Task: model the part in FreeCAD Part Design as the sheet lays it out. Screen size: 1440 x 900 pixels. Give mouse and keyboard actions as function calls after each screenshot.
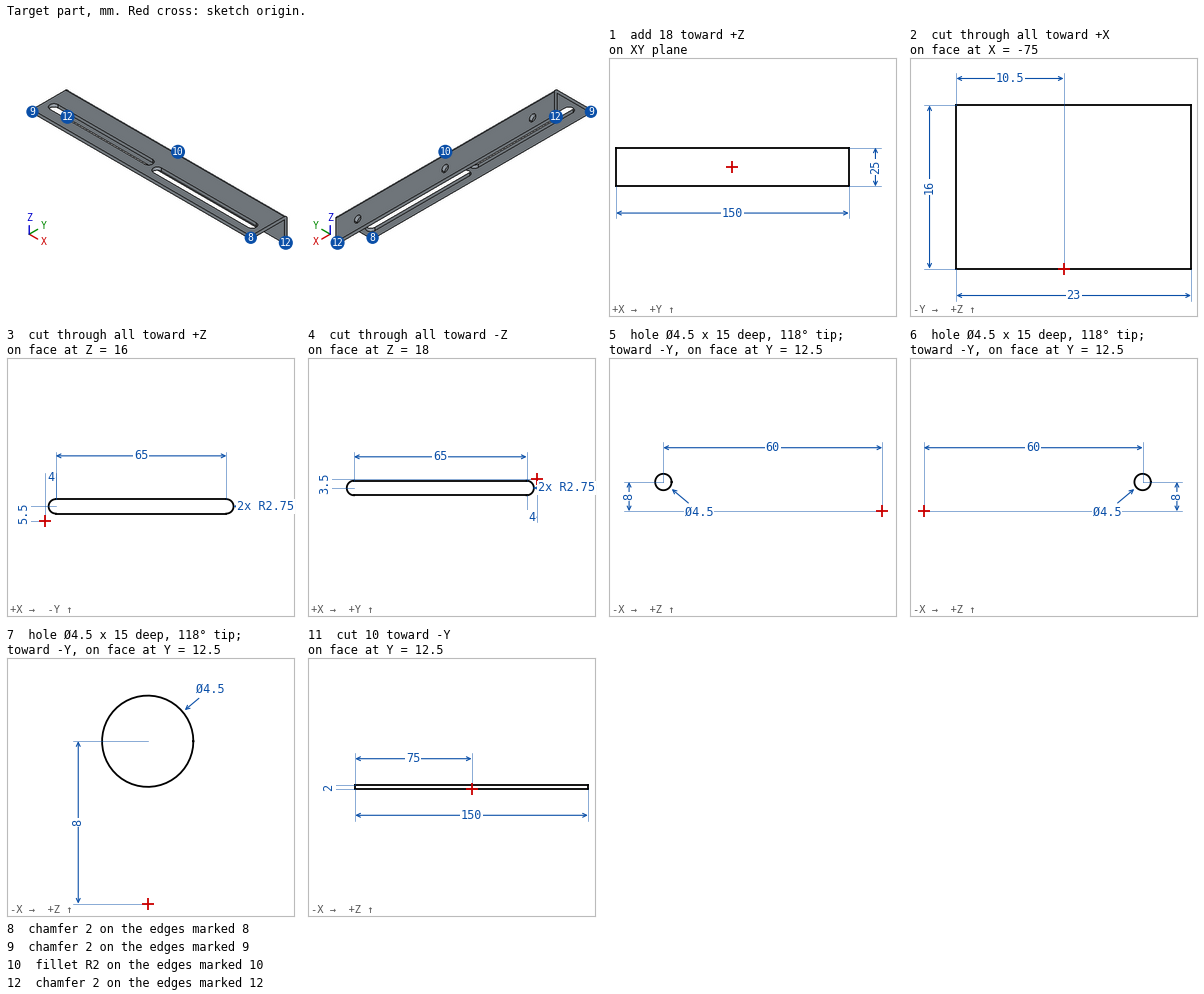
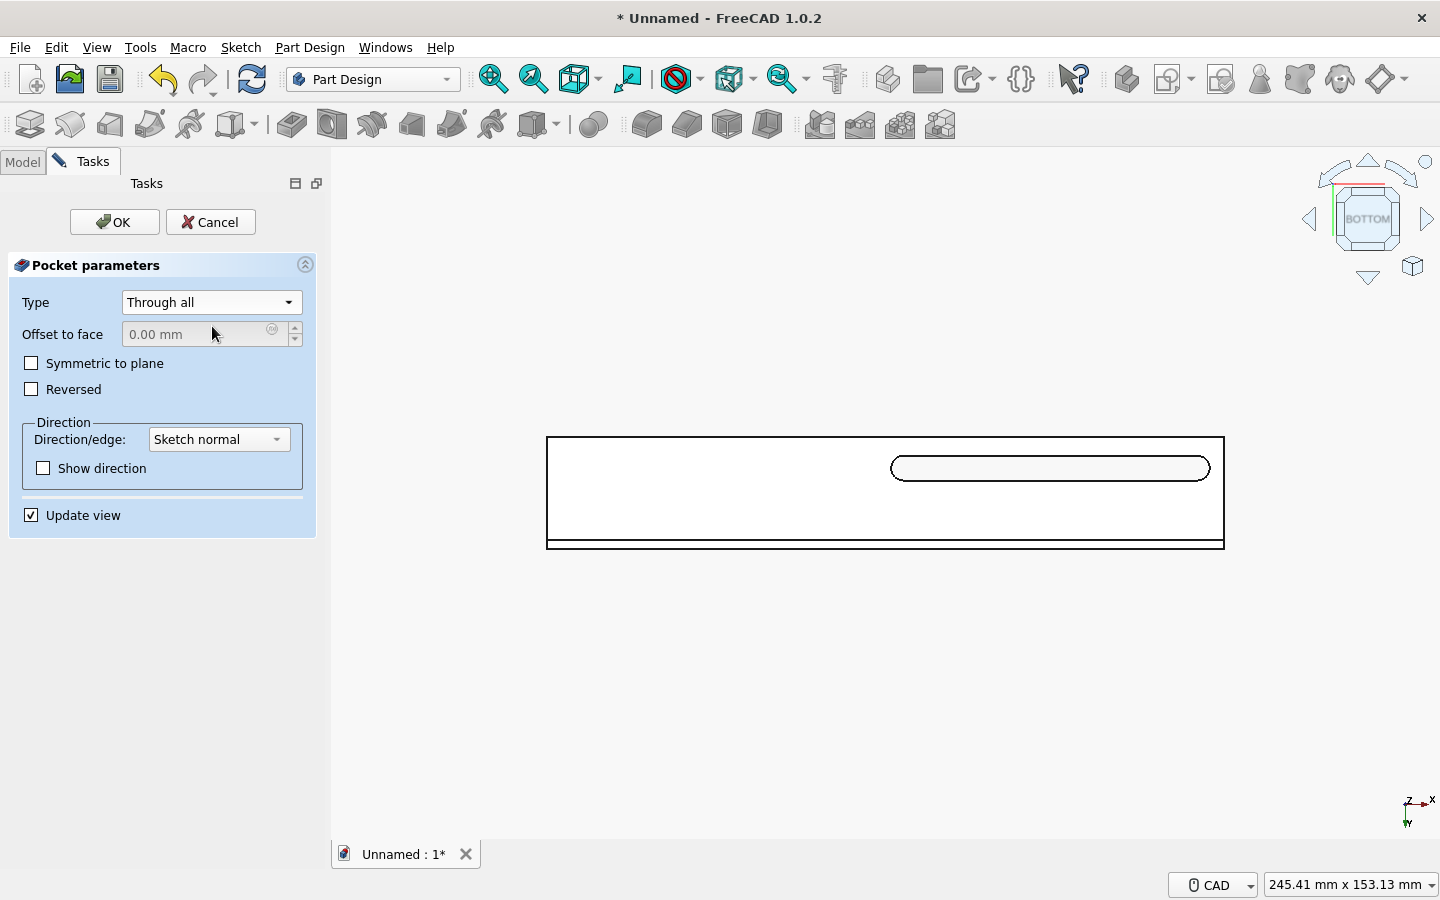
click(115, 222)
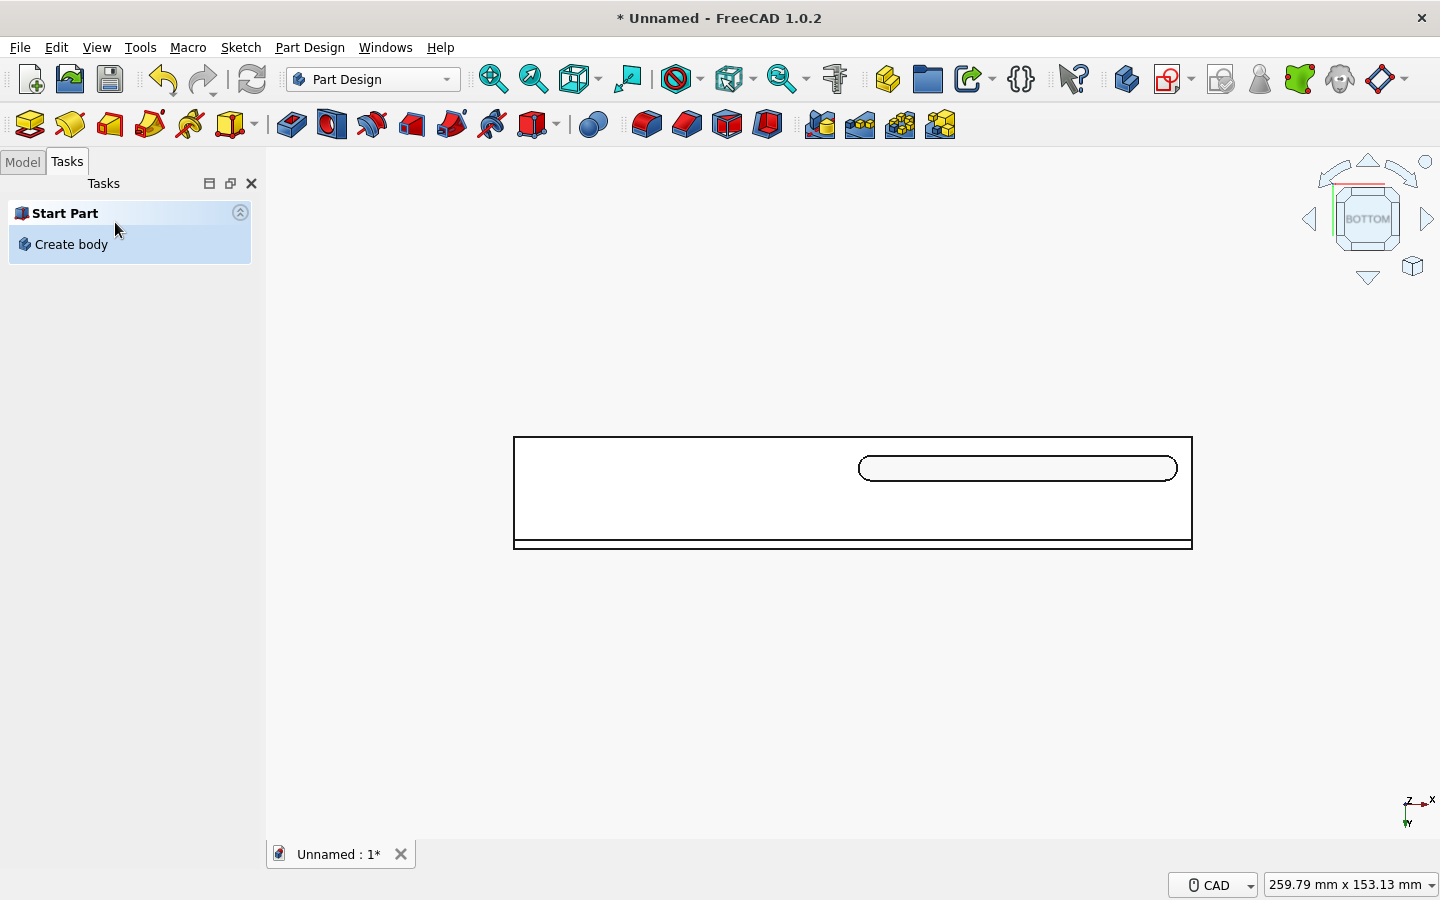
key(0)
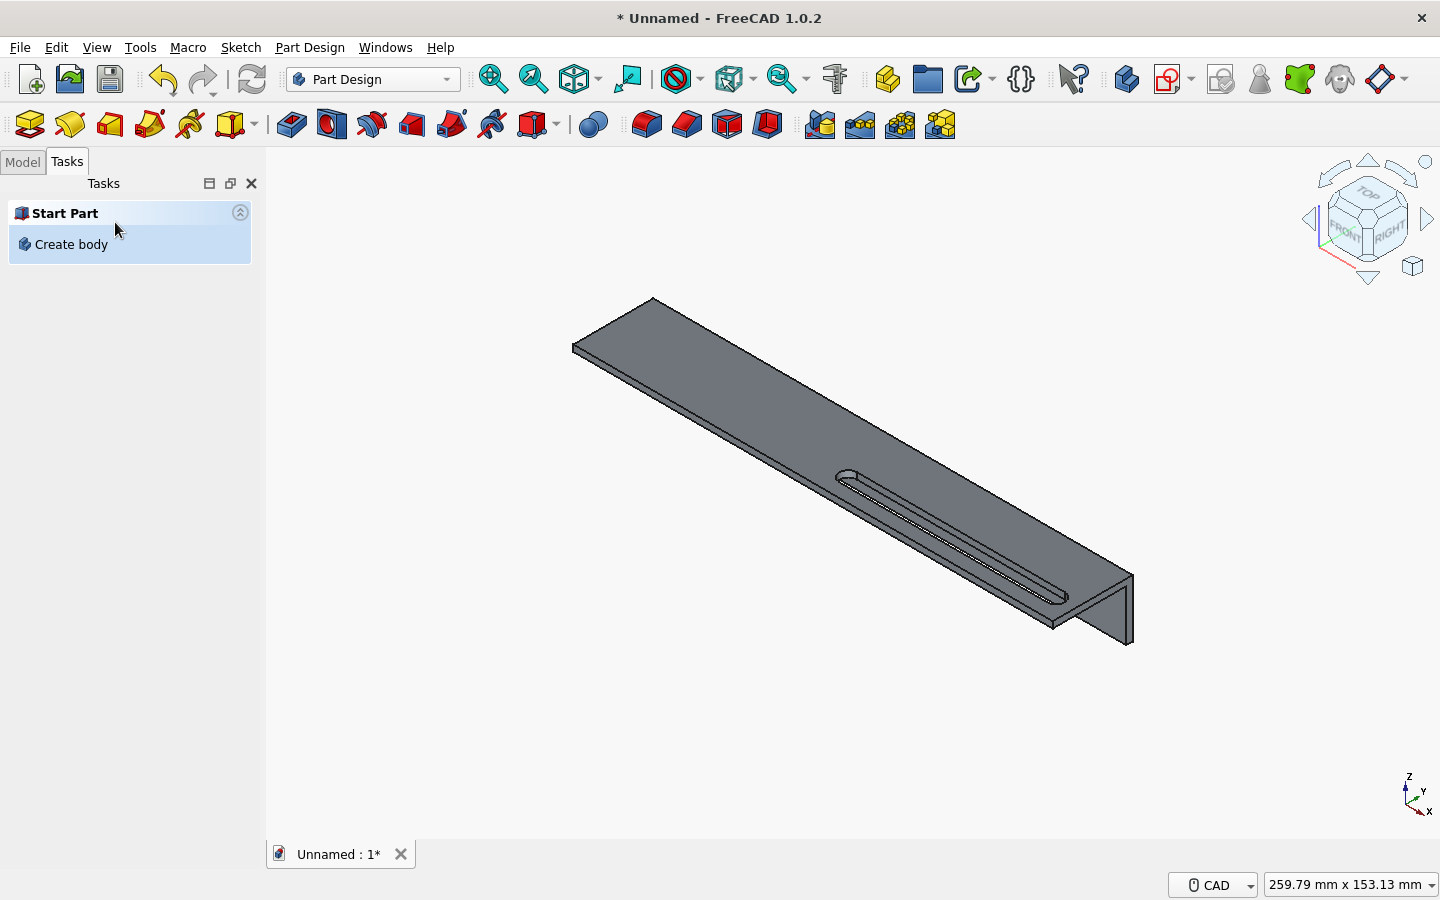
click(785, 419)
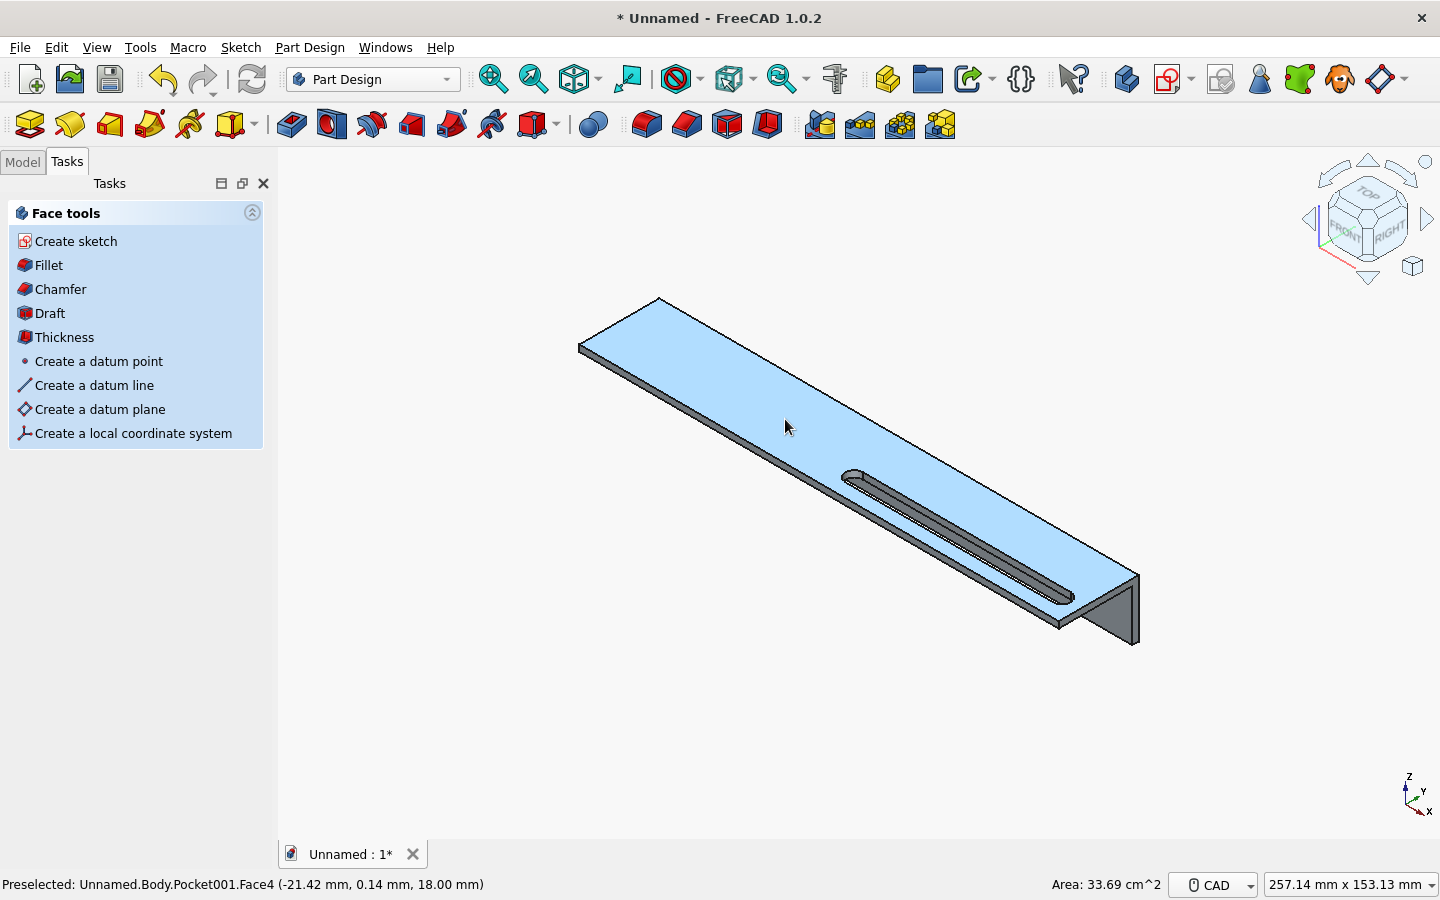
click(1168, 80)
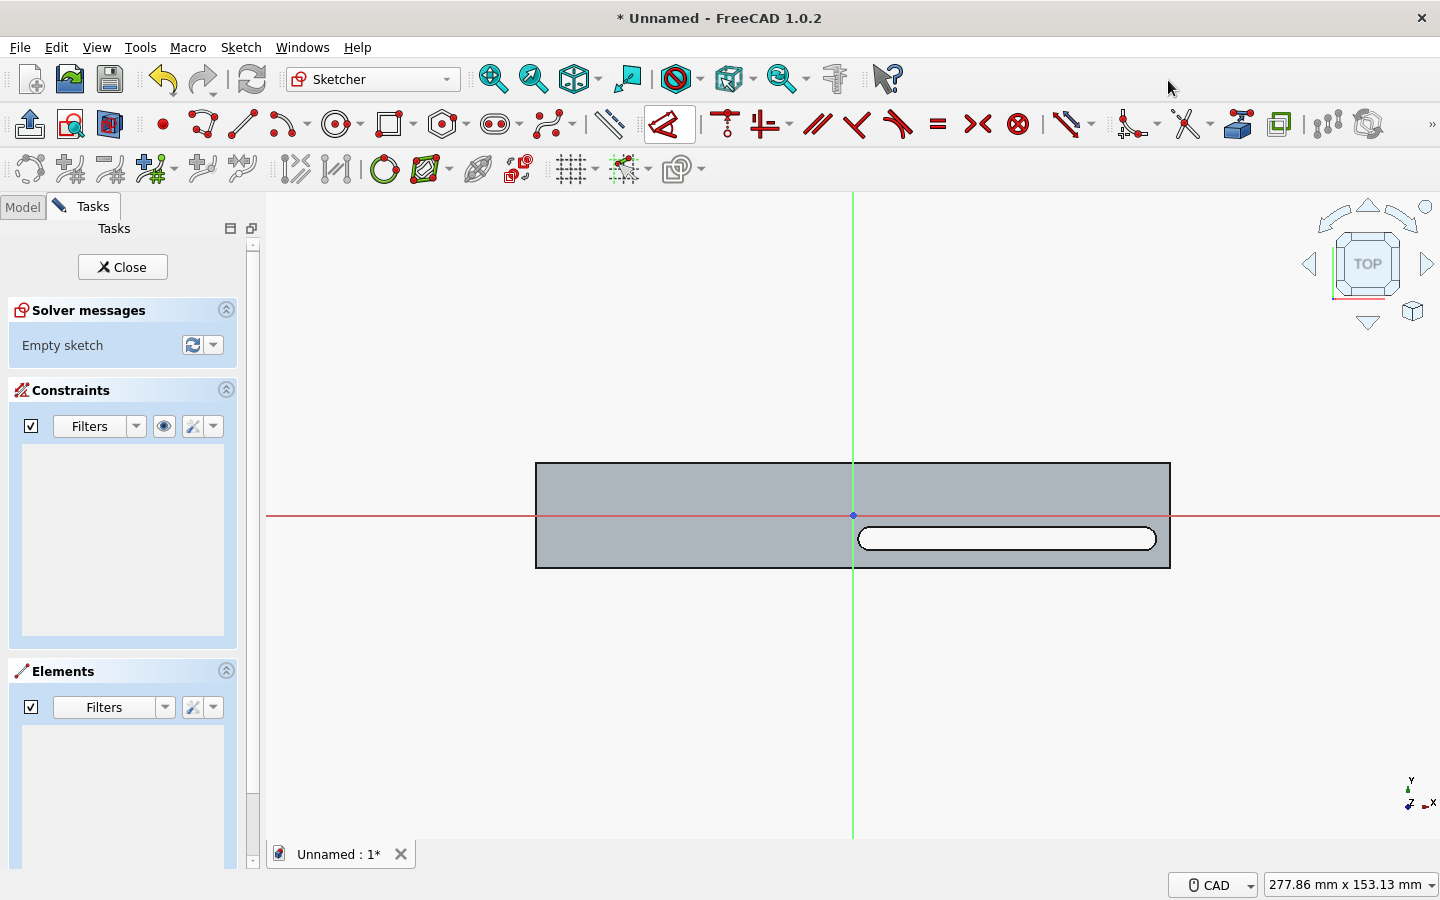
scroll(634, 539, up, 4)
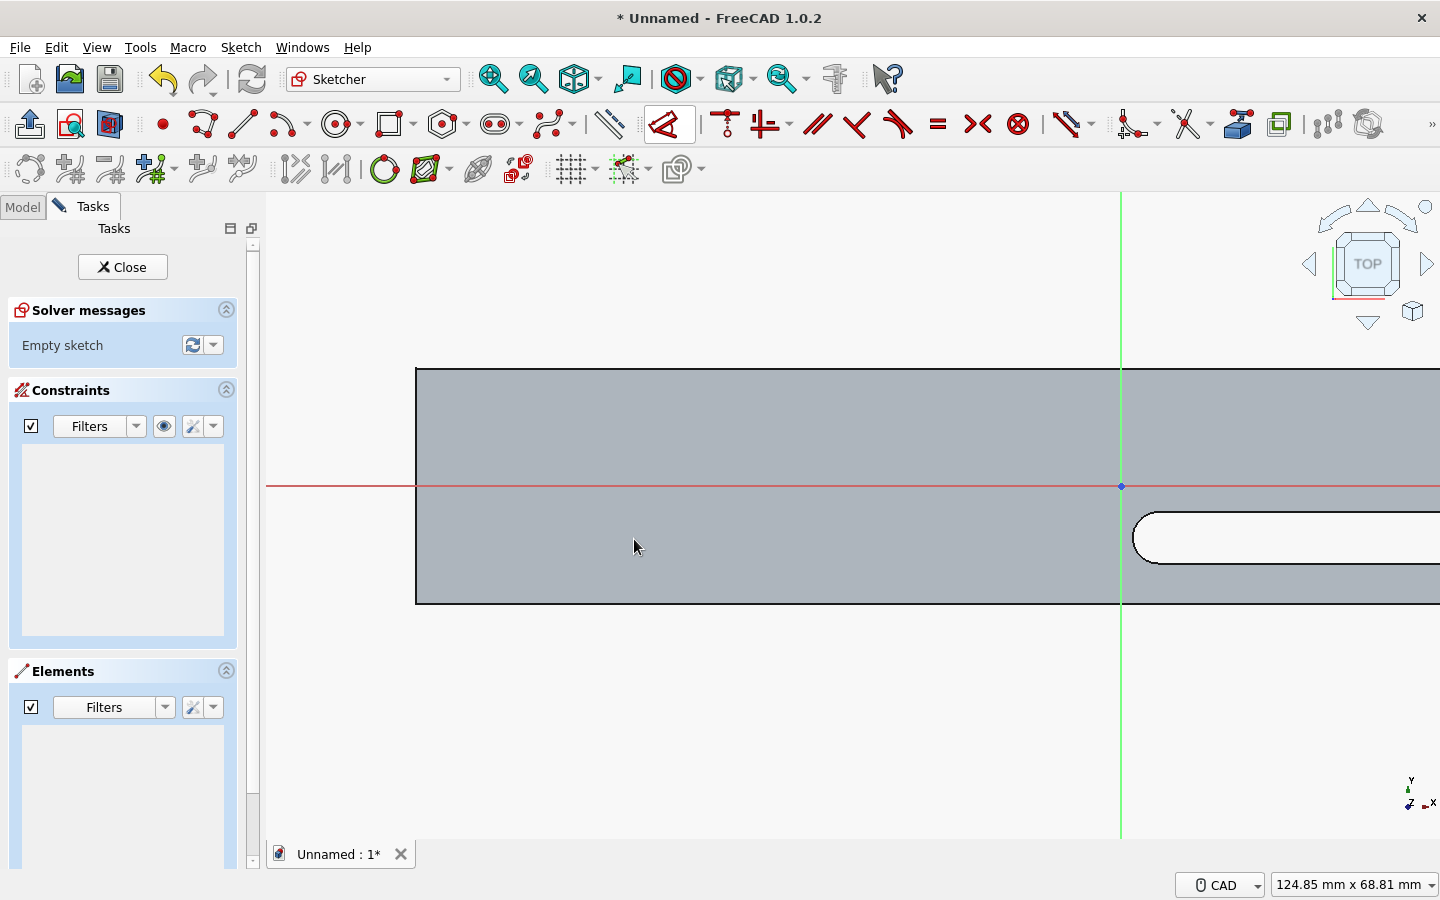
click(496, 124)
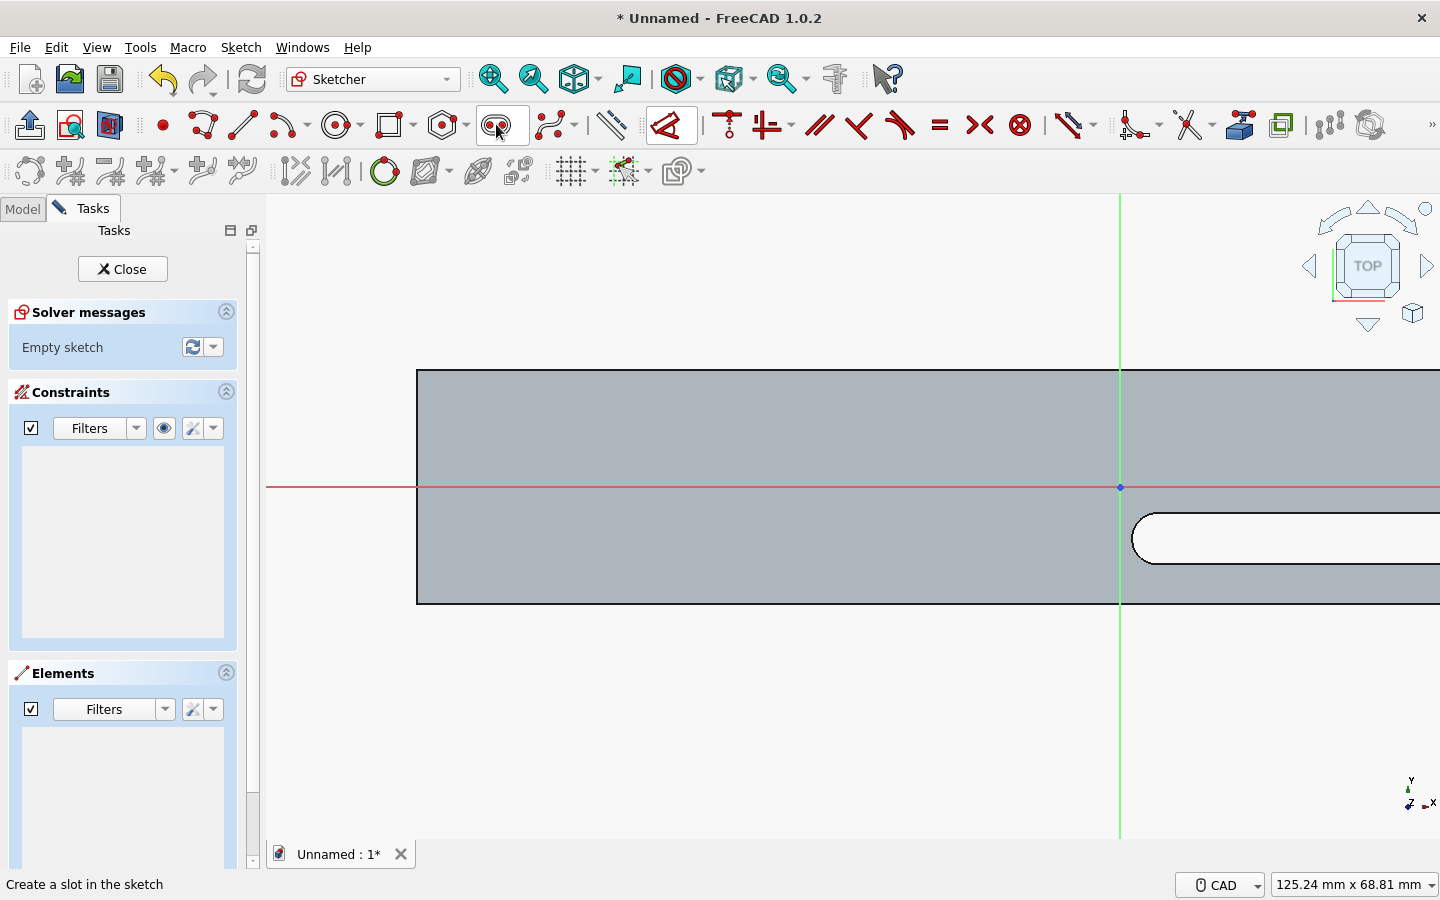
click(473, 520)